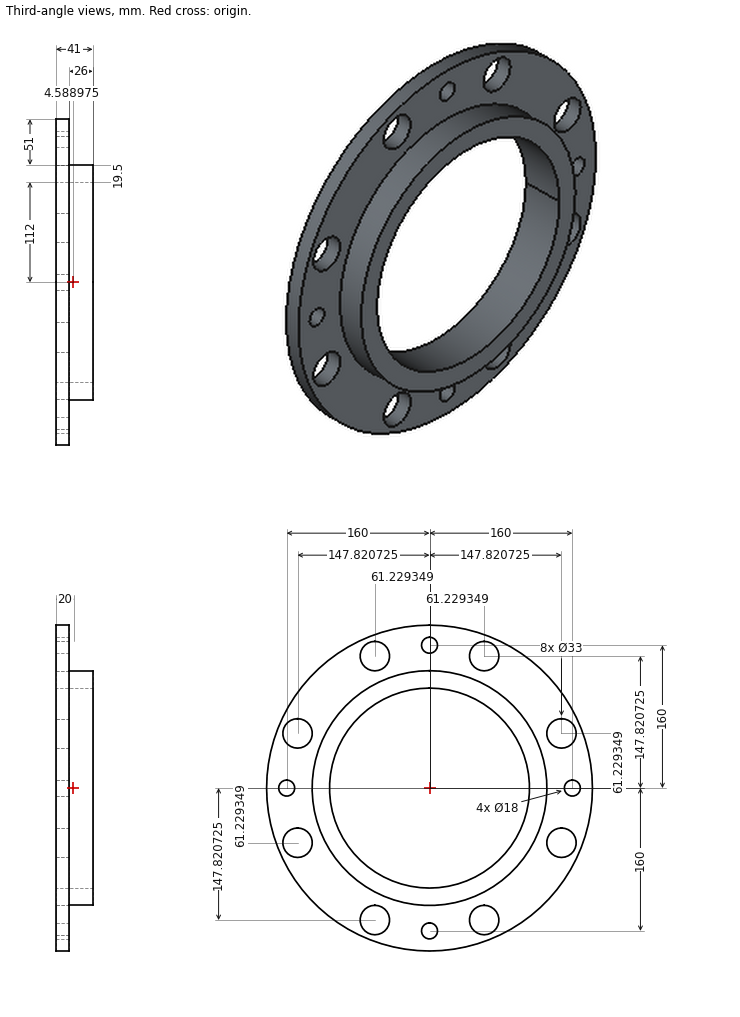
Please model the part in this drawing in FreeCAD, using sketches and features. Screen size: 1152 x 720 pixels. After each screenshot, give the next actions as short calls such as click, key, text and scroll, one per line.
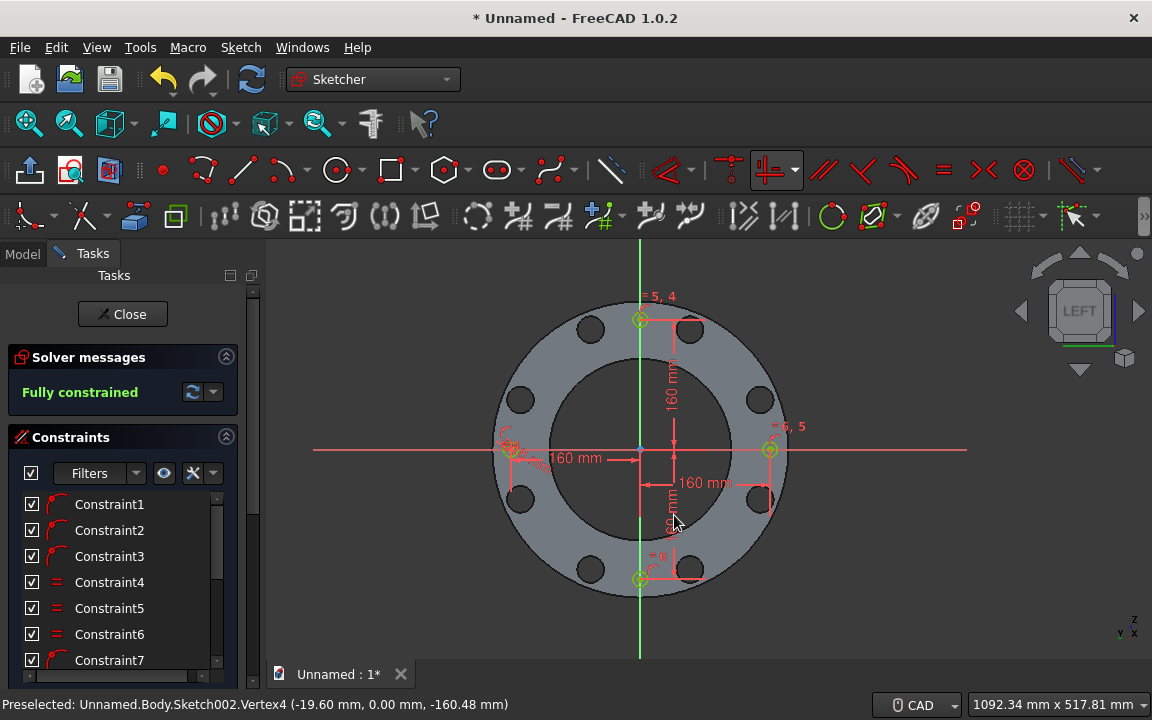
click(123, 314)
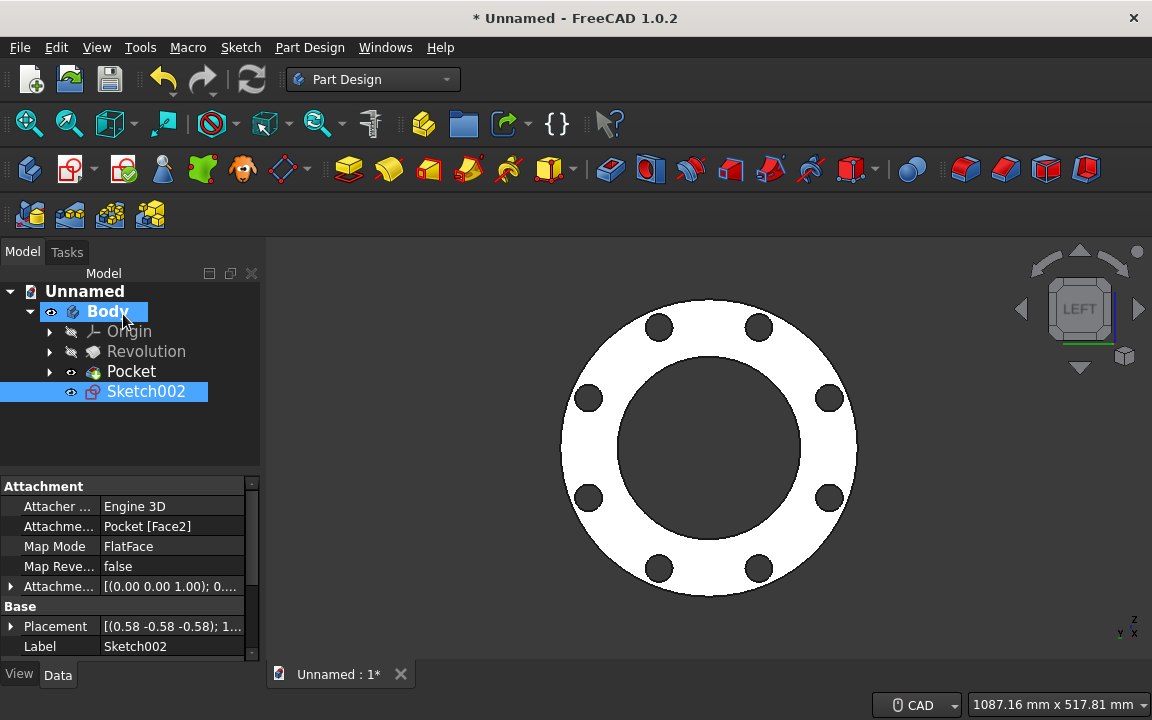
click(612, 170)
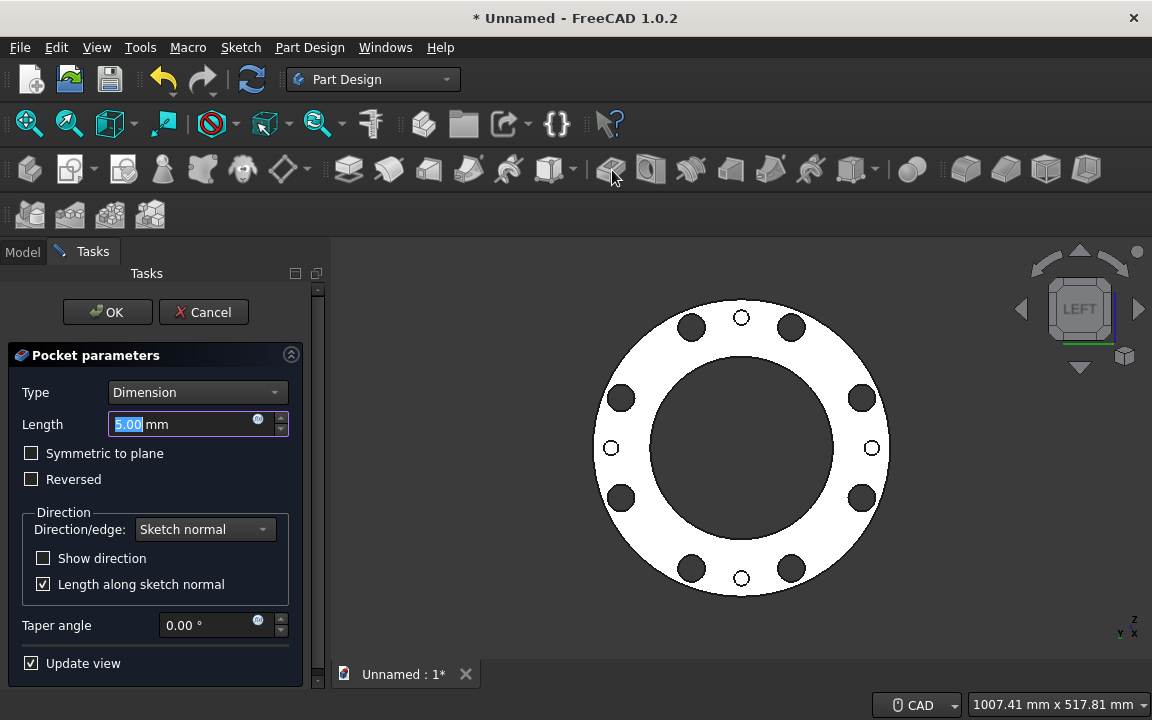
text(20)
key(Tab)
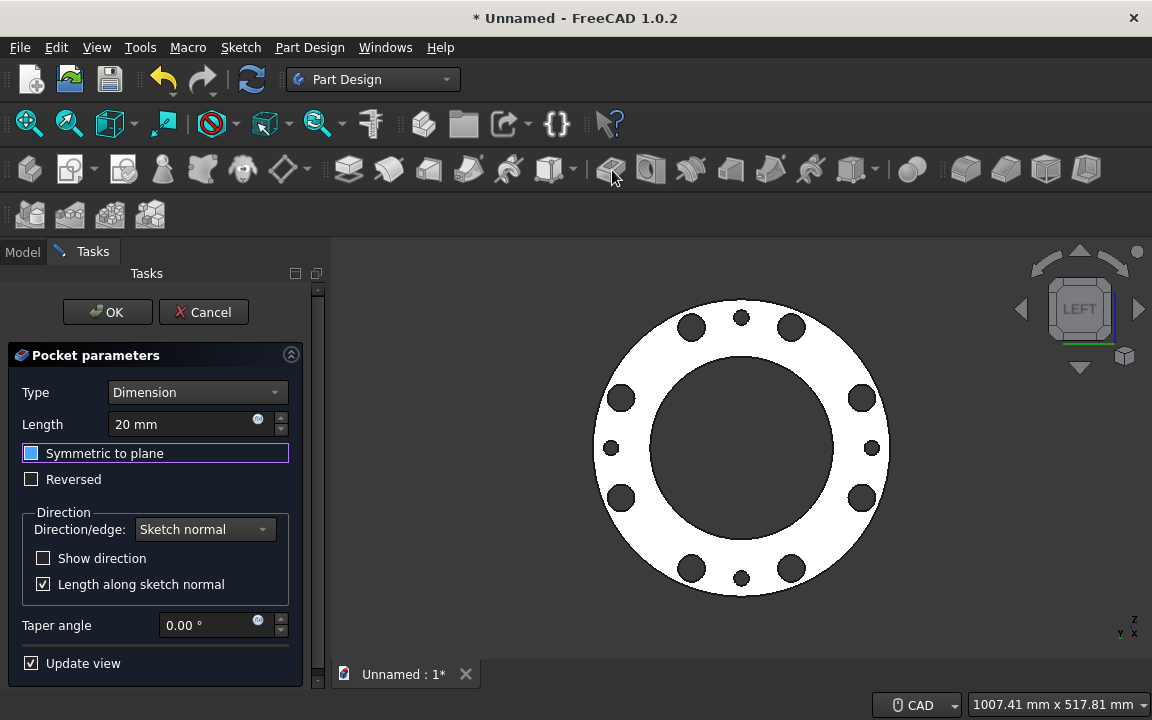
click(108, 312)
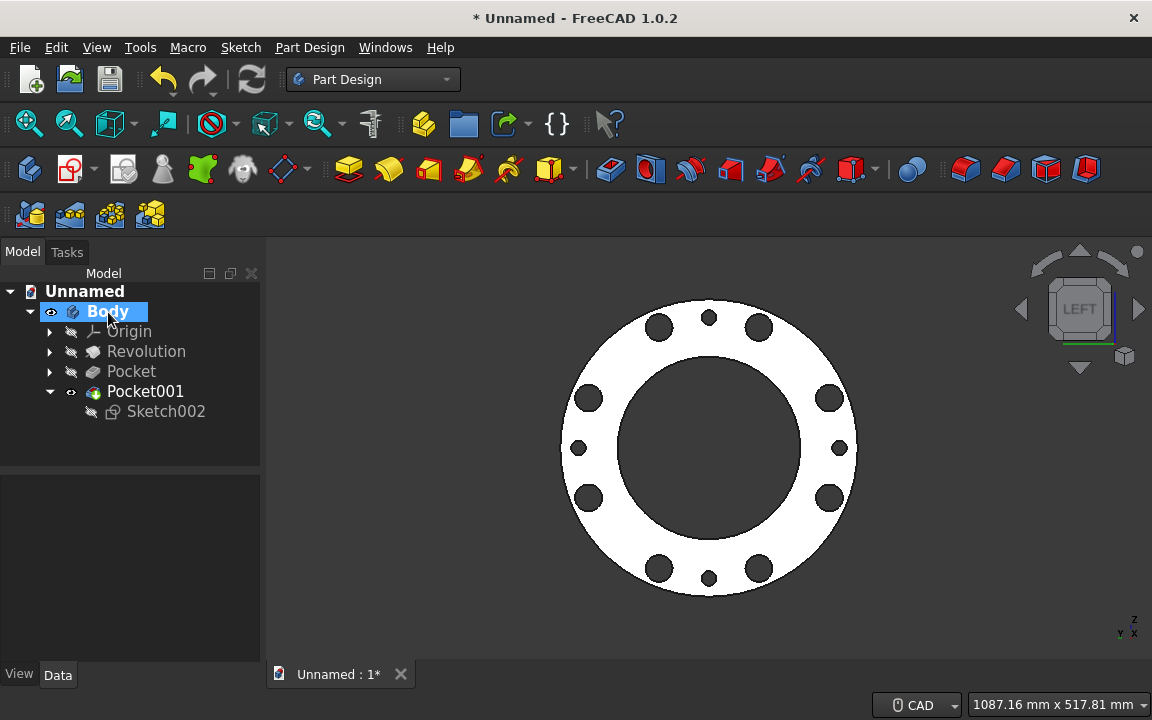
key(0)